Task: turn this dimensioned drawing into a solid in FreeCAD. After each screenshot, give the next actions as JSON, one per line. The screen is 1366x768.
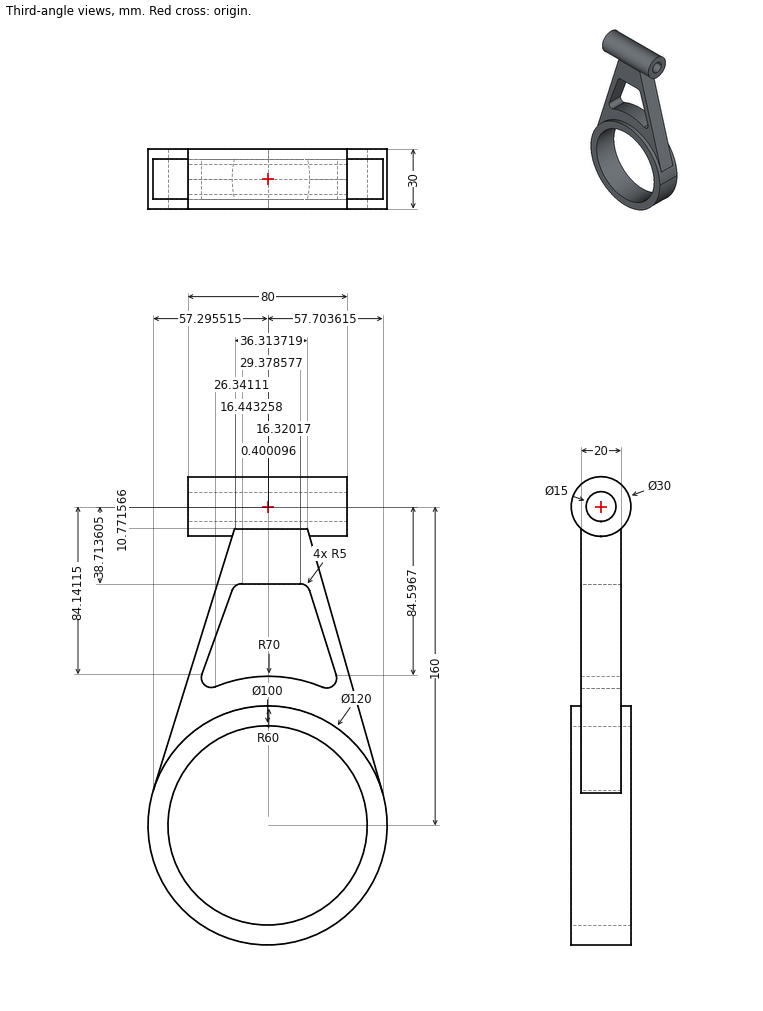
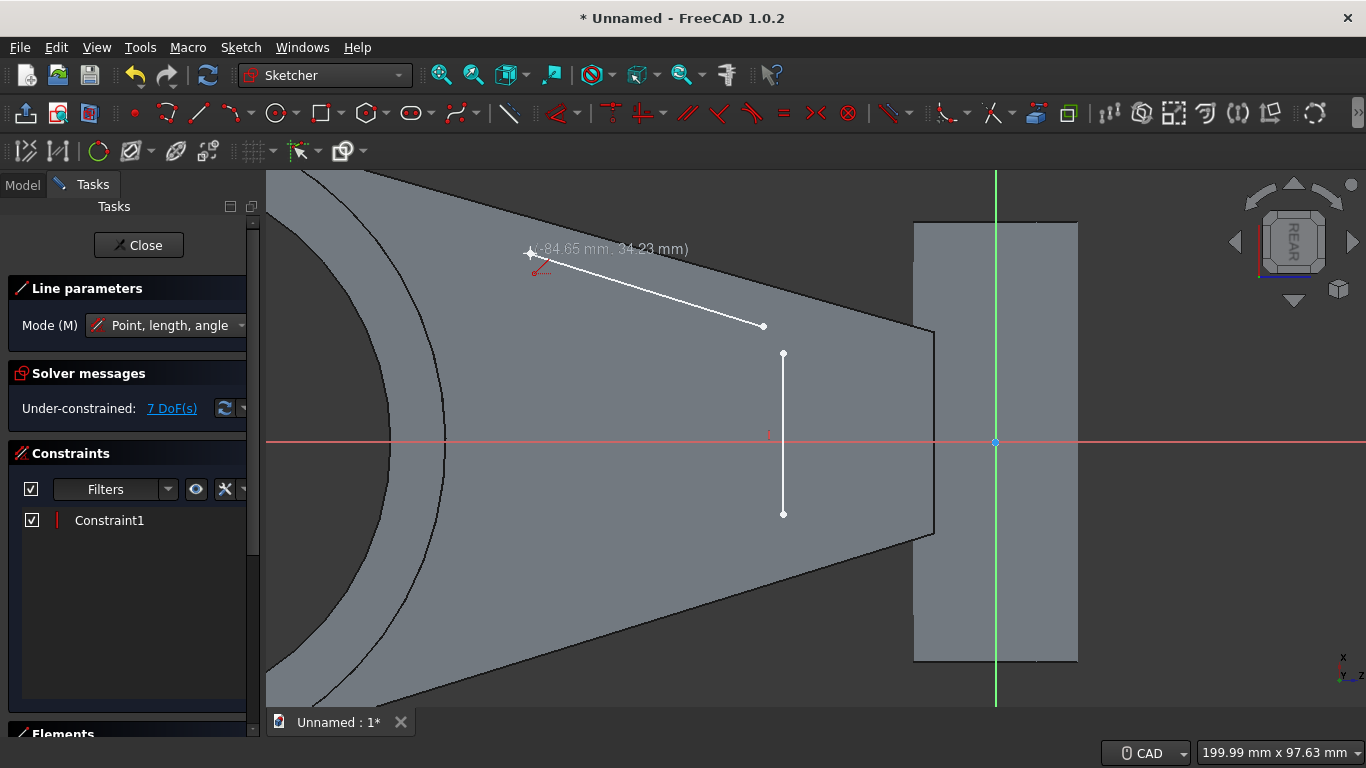
{"action": "left_click", "coordinate": [533, 624]}
{"action": "left_click", "coordinate": [765, 540]}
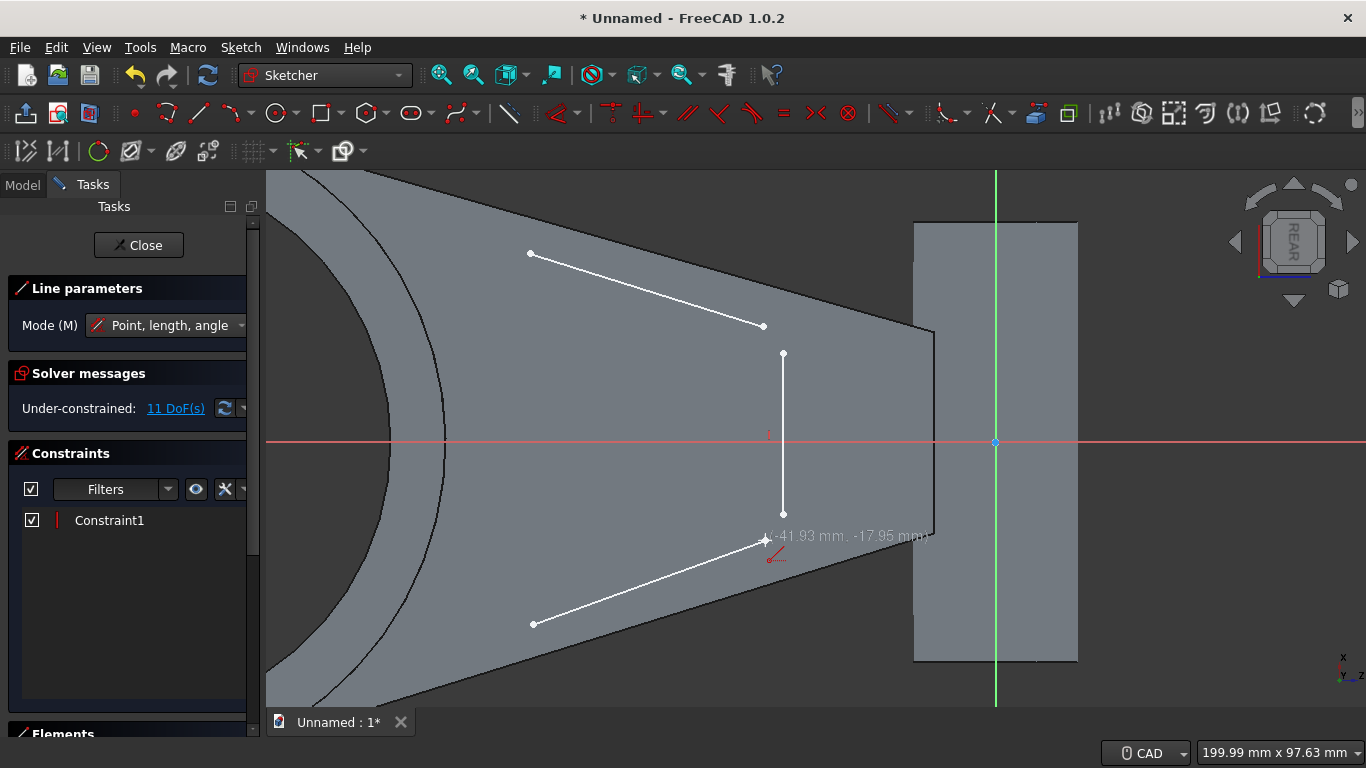
{"action": "left_click", "coordinate": [232, 114]}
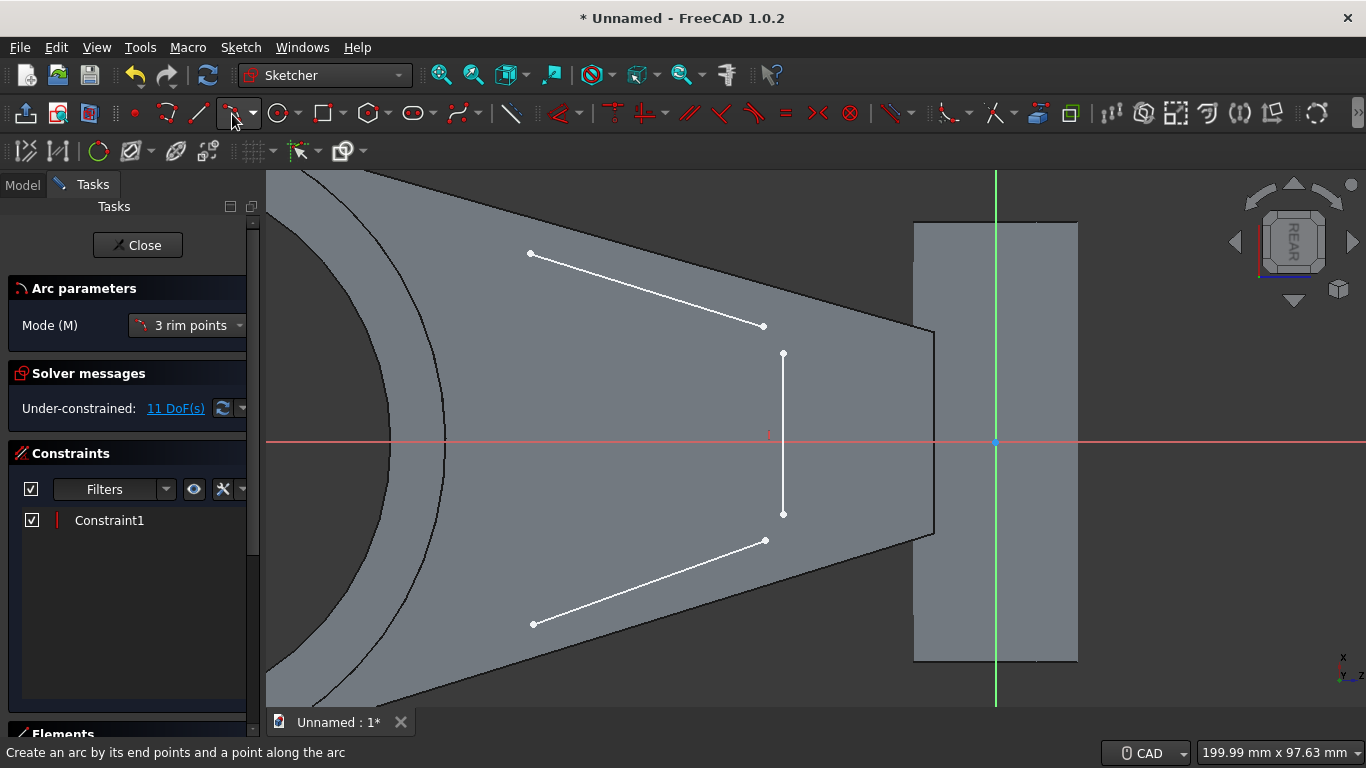
{"action": "left_click", "coordinate": [783, 354]}
{"action": "left_click", "coordinate": [763, 327]}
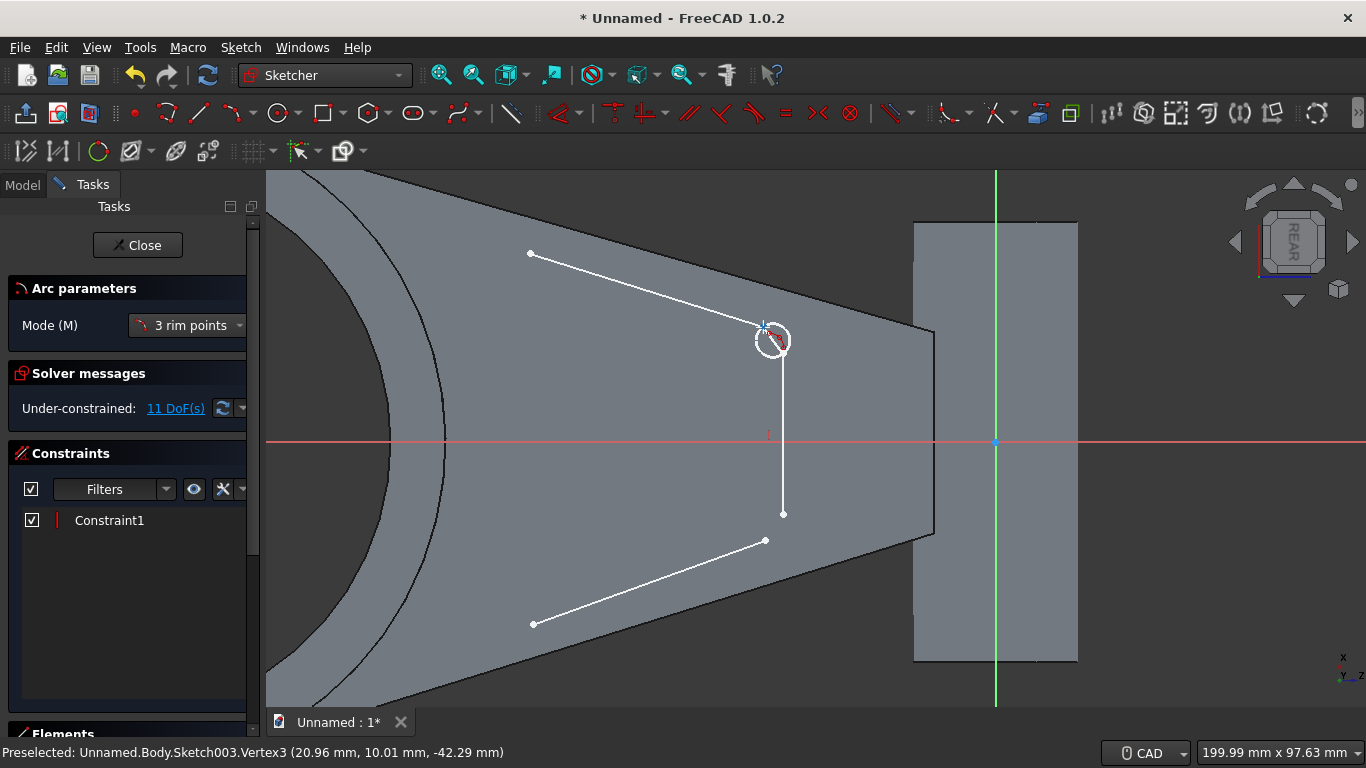
{"action": "scroll", "coordinate": [777, 336], "scroll_direction": "up", "scroll_amount": 6}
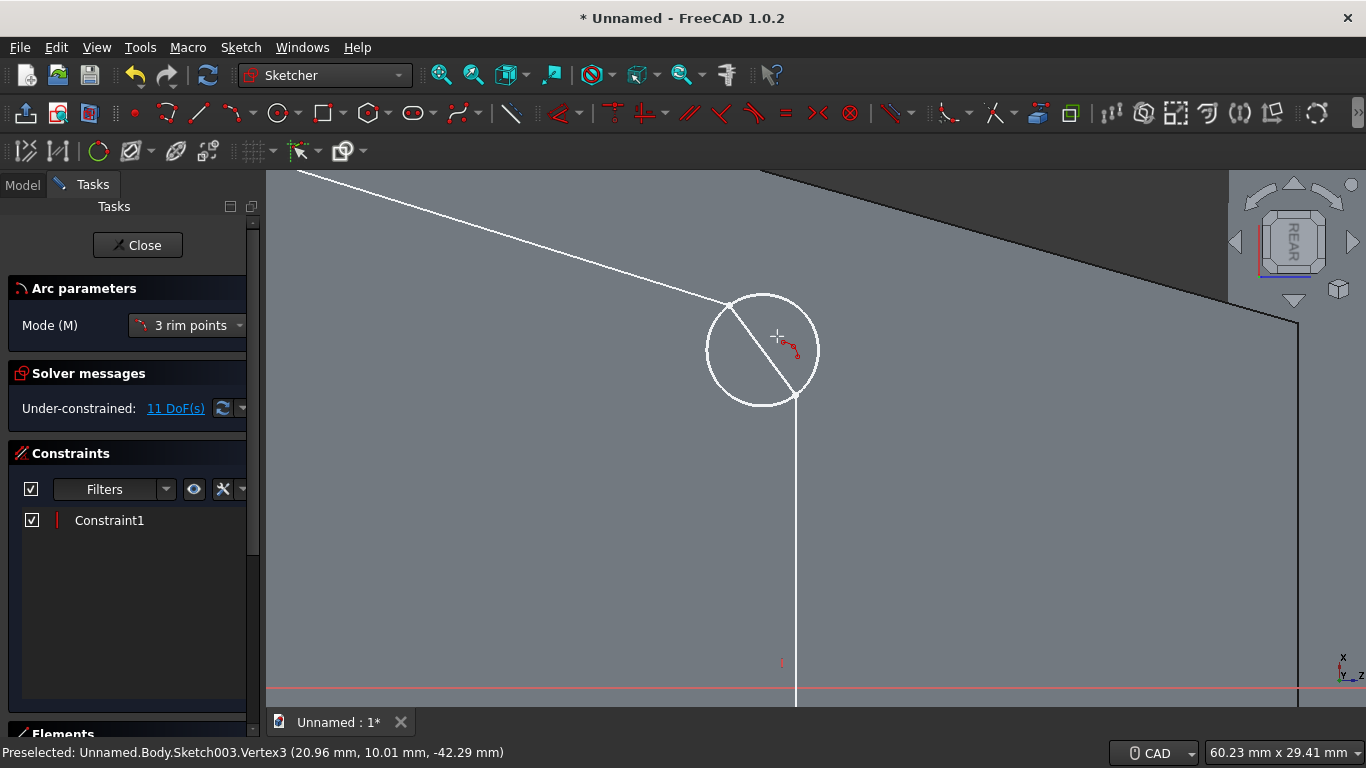
{"action": "left_click", "coordinate": [777, 336]}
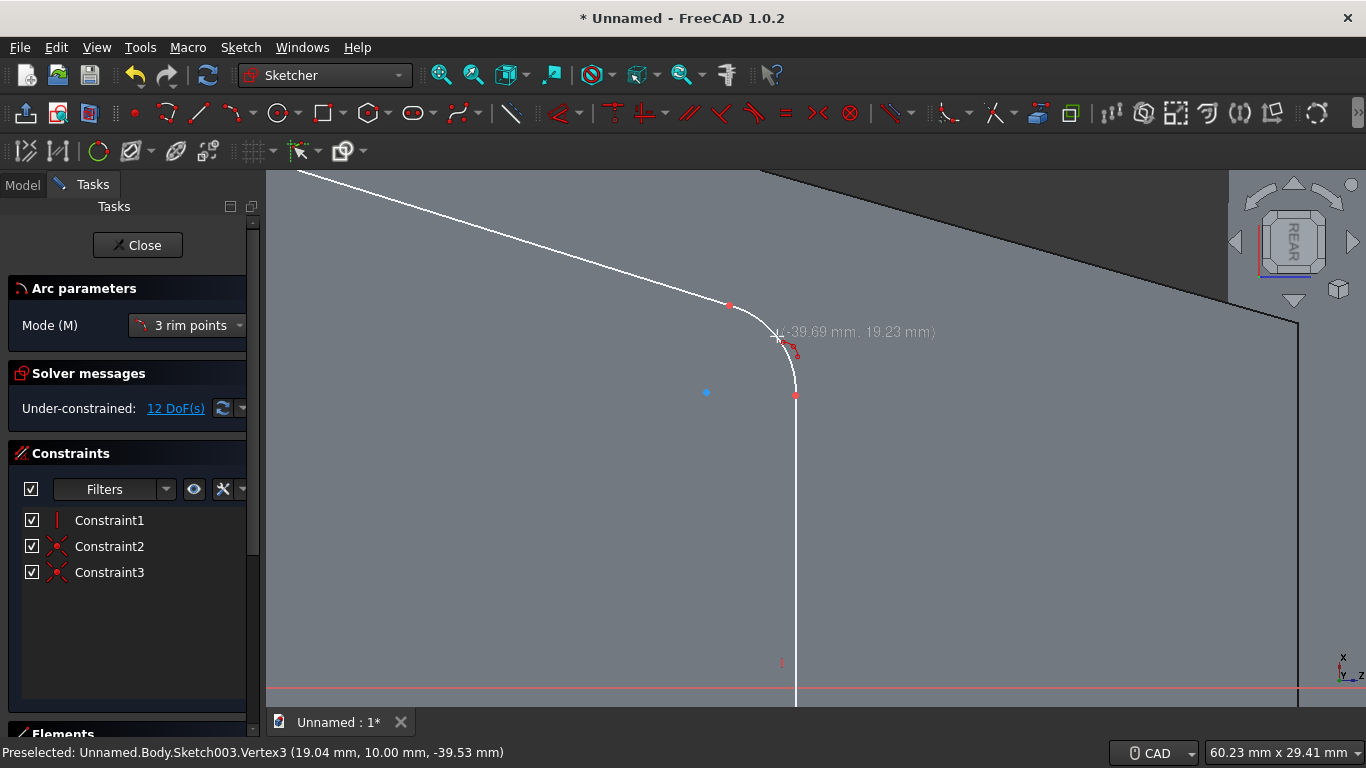
{"action": "scroll", "coordinate": [779, 337], "scroll_direction": "down", "scroll_amount": 6}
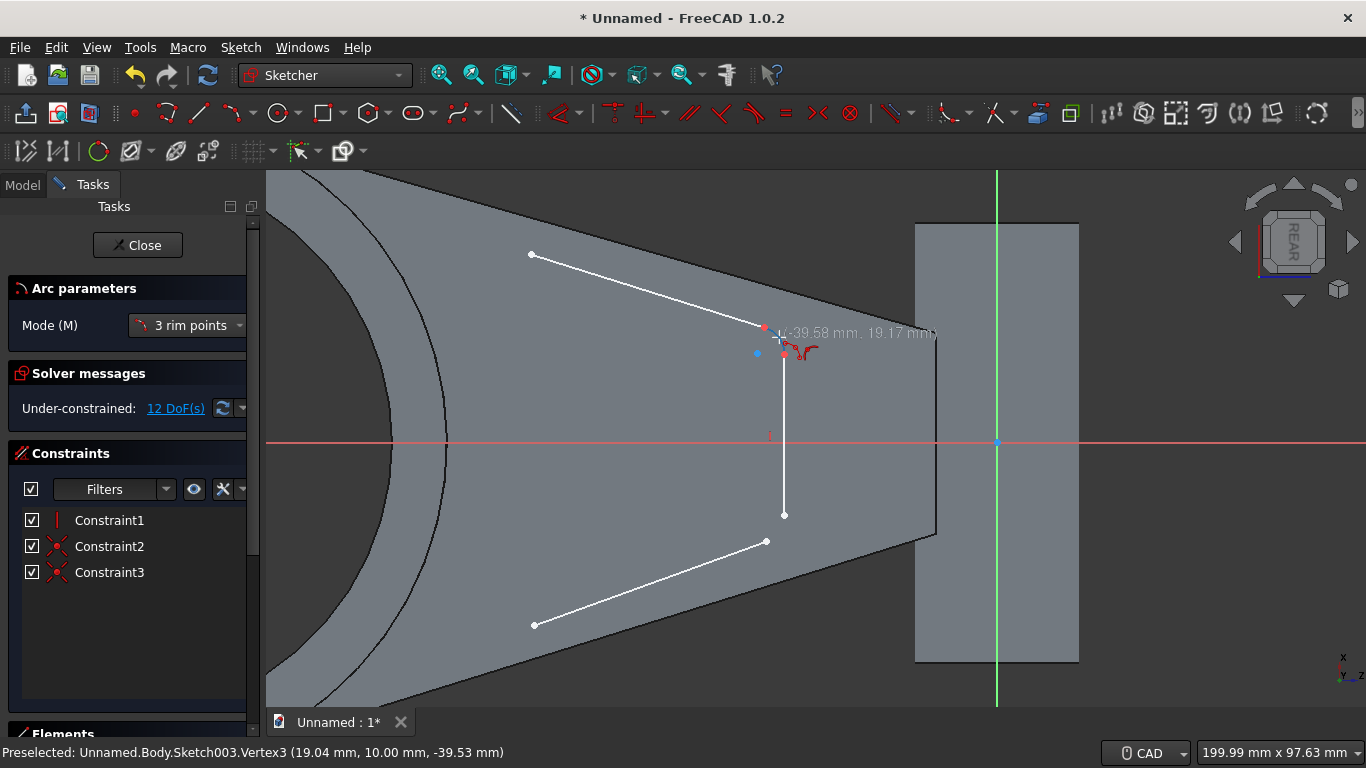
{"action": "left_click", "coordinate": [531, 255]}
{"action": "left_click", "coordinate": [498, 290]}
{"action": "left_click", "coordinate": [503, 261]}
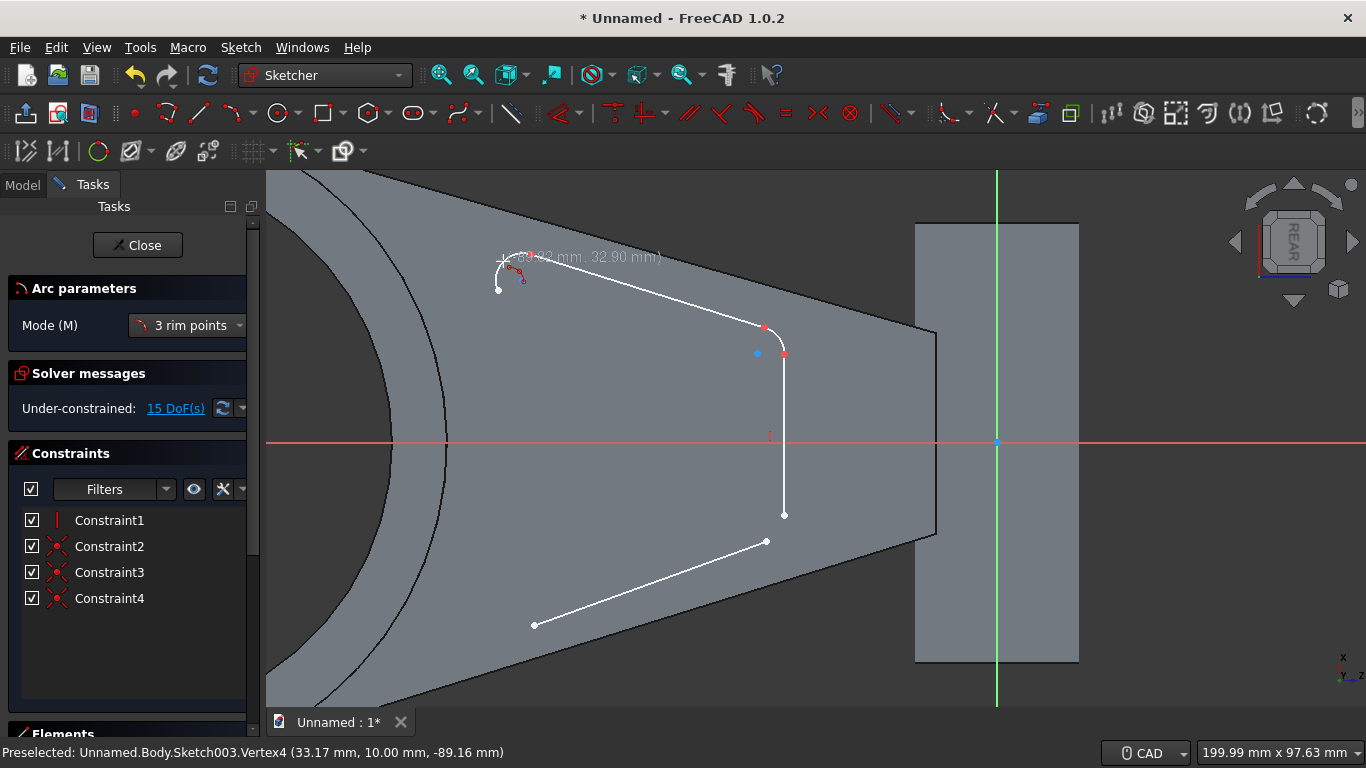
{"action": "left_click", "coordinate": [498, 291]}
{"action": "left_click", "coordinate": [499, 588]}
{"action": "left_click", "coordinate": [528, 470]}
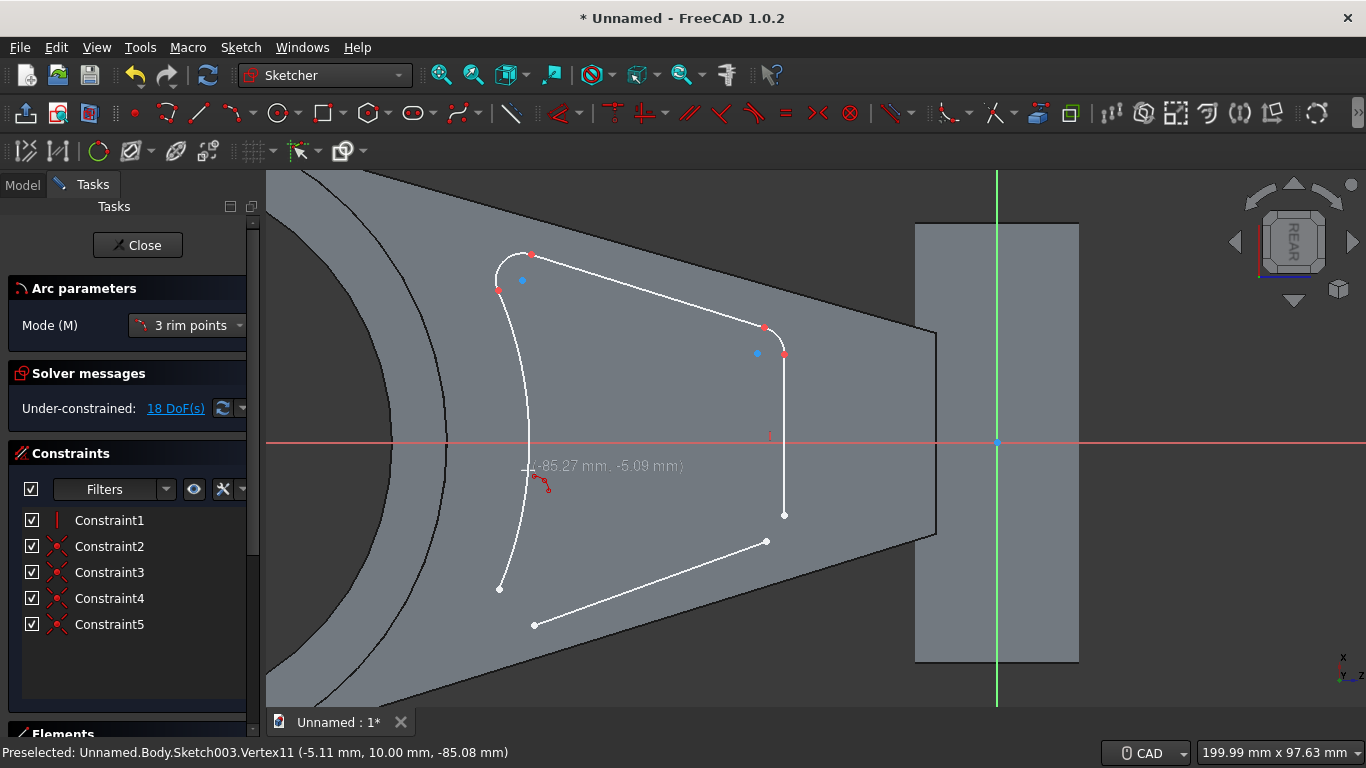
{"action": "left_click", "coordinate": [499, 589]}
{"action": "left_click", "coordinate": [534, 626]}
{"action": "left_click", "coordinate": [505, 617]}